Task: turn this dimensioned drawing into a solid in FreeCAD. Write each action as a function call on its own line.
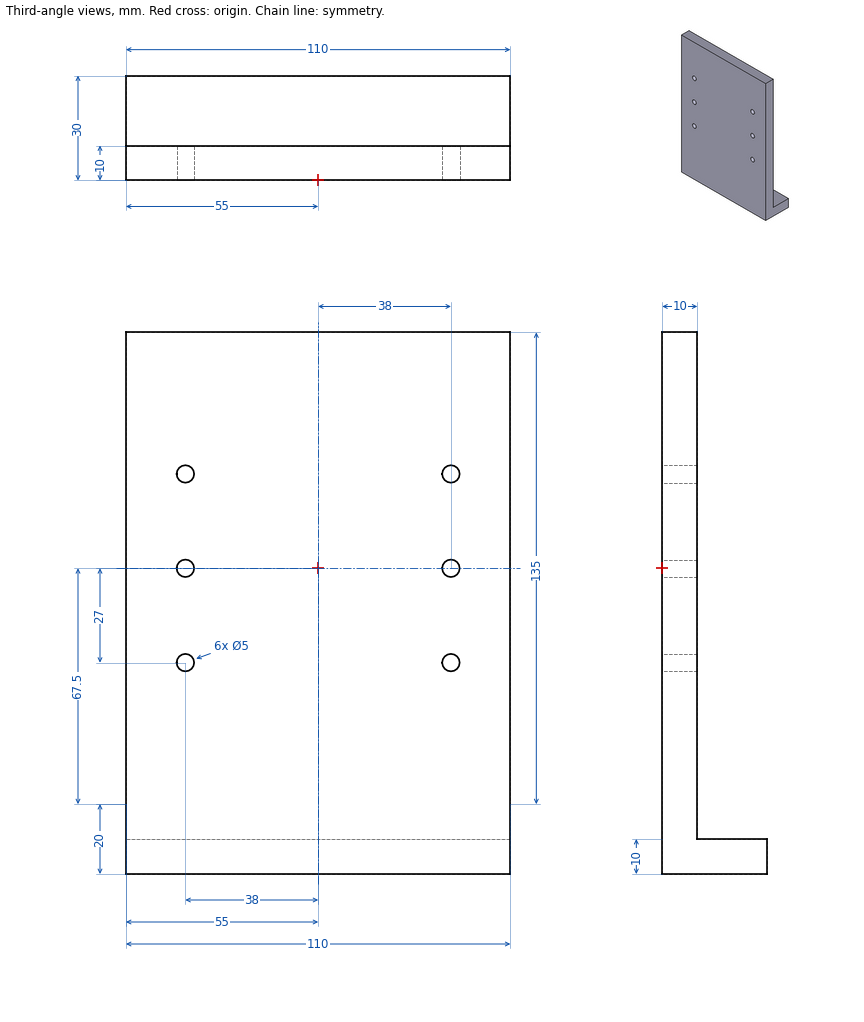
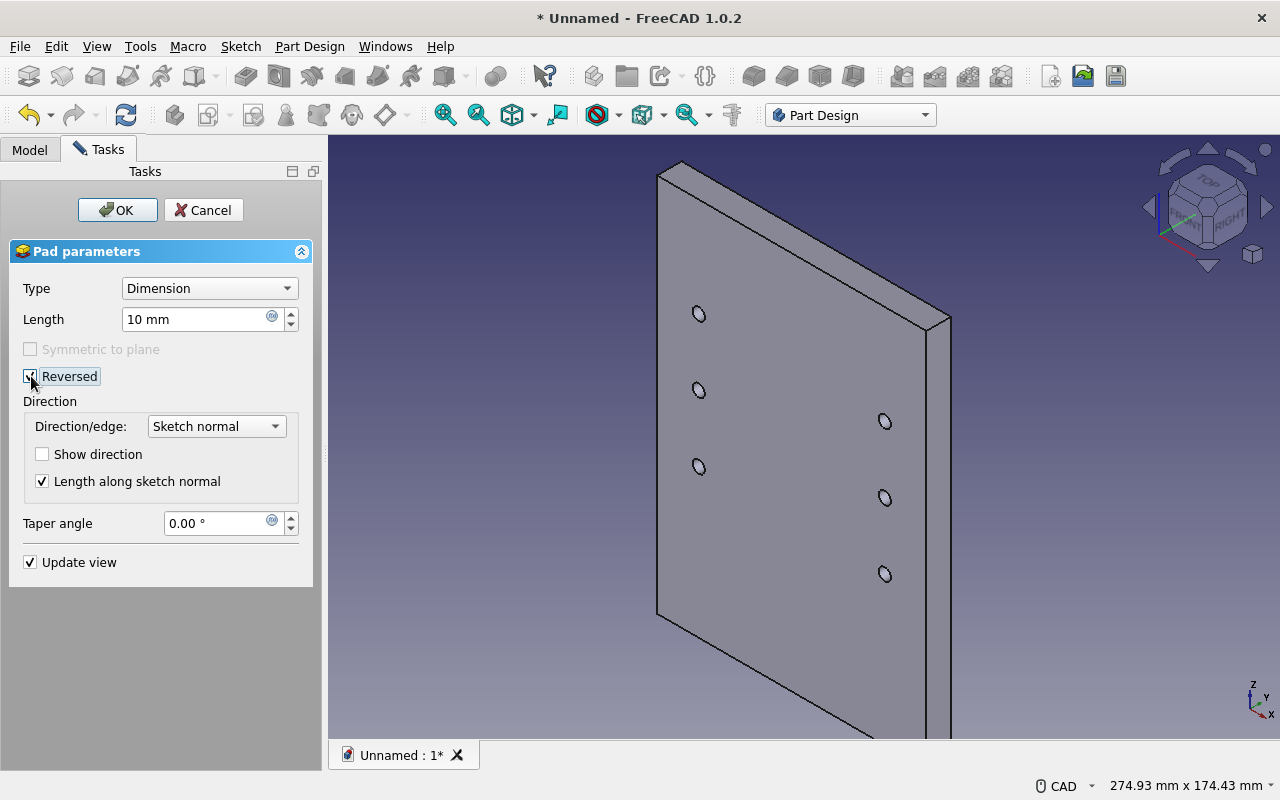
click(118, 210)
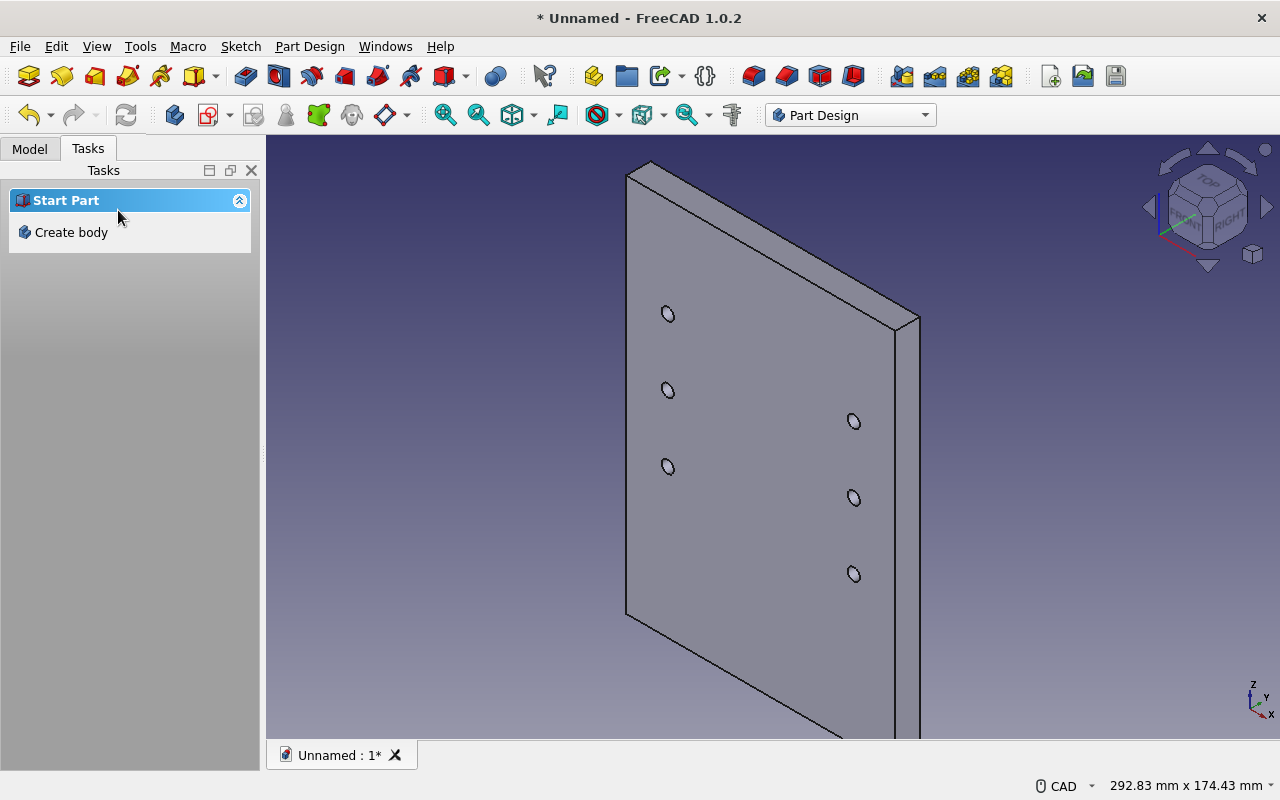
click(446, 116)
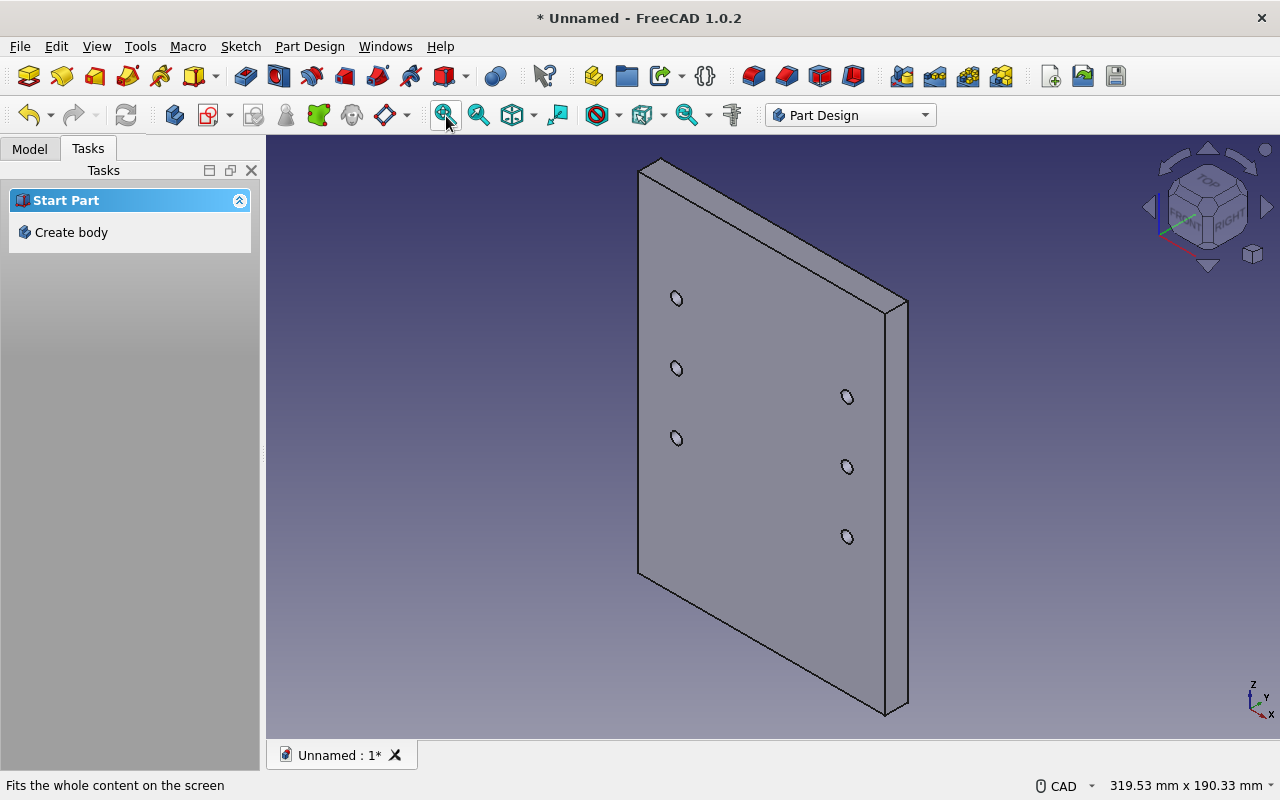
key(5)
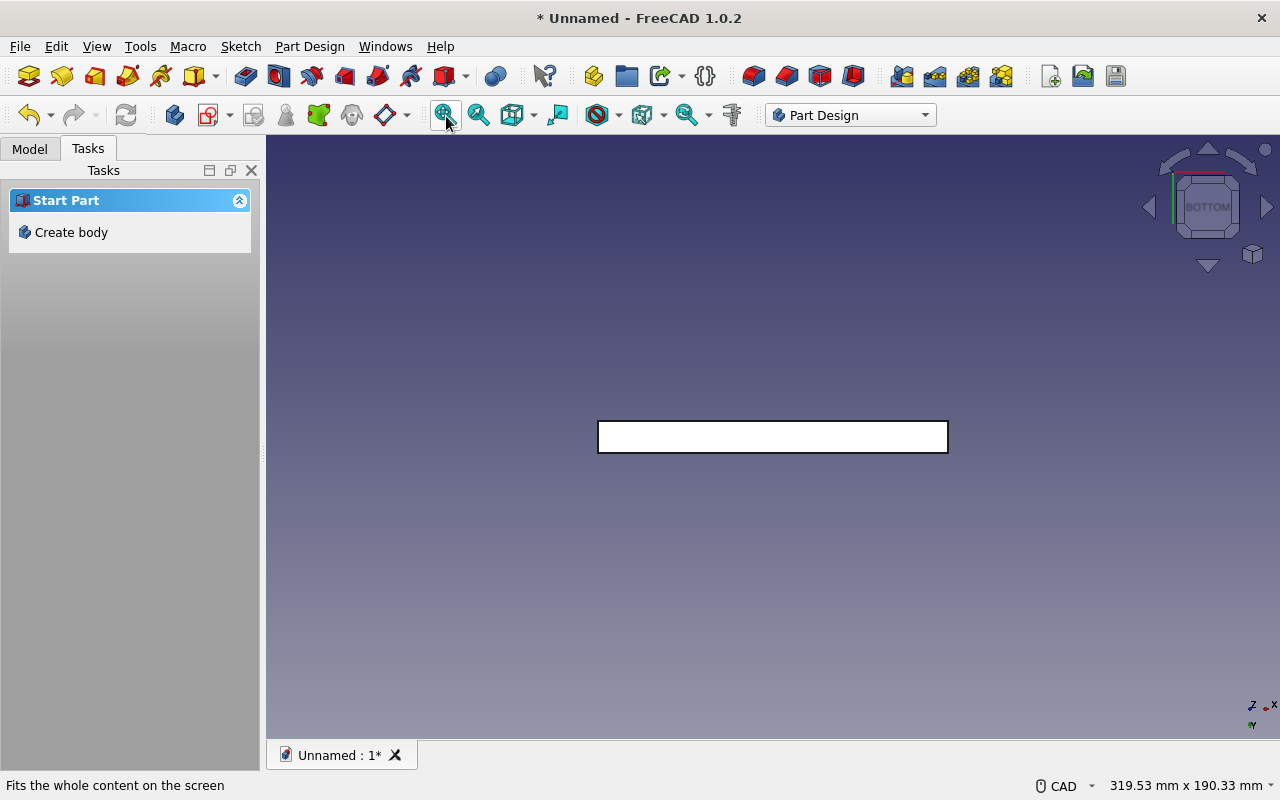
click(446, 116)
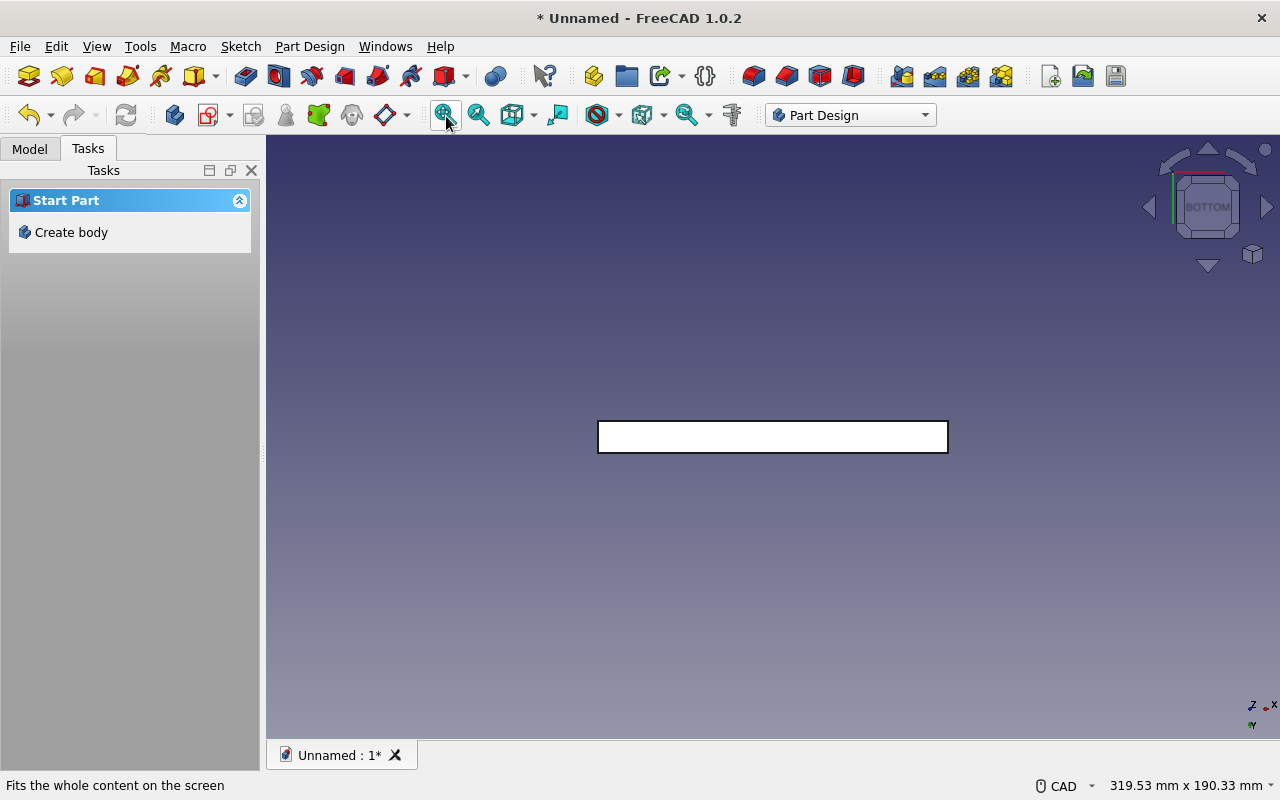
click(923, 436)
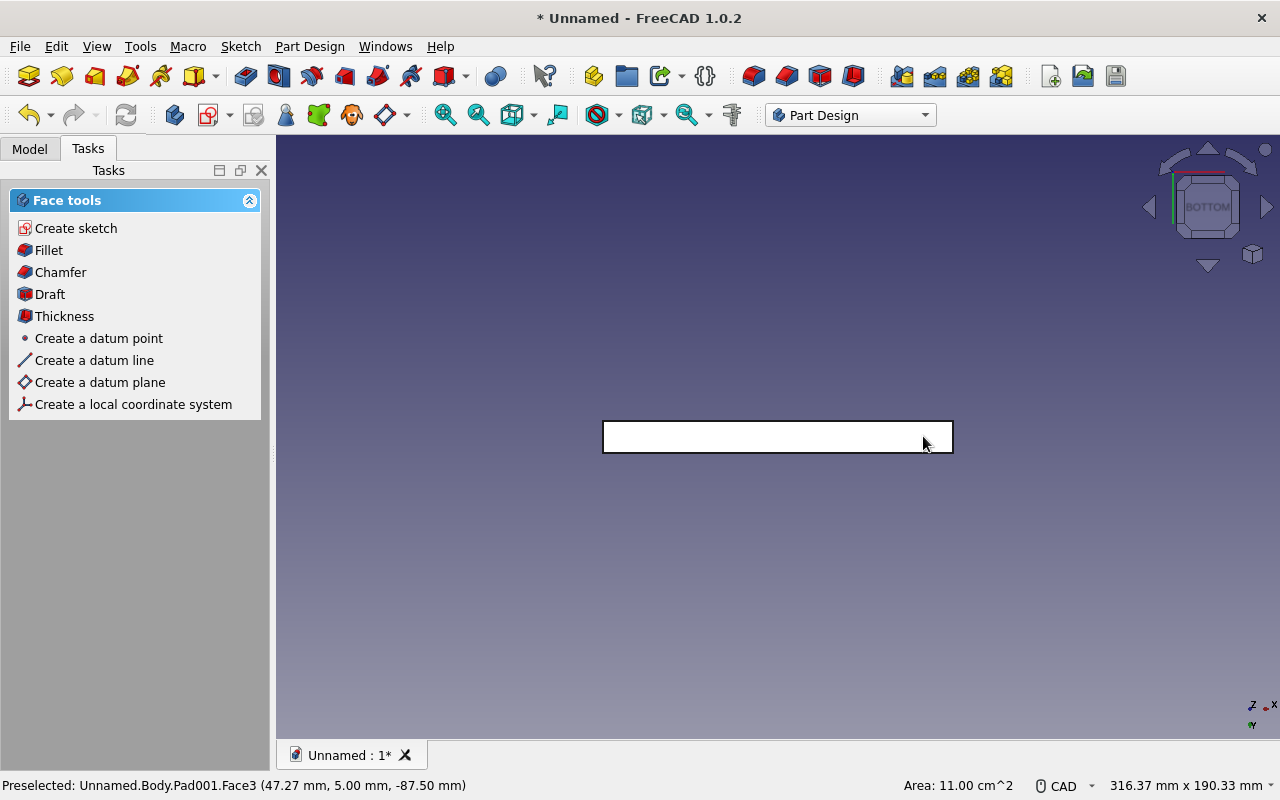
click(208, 116)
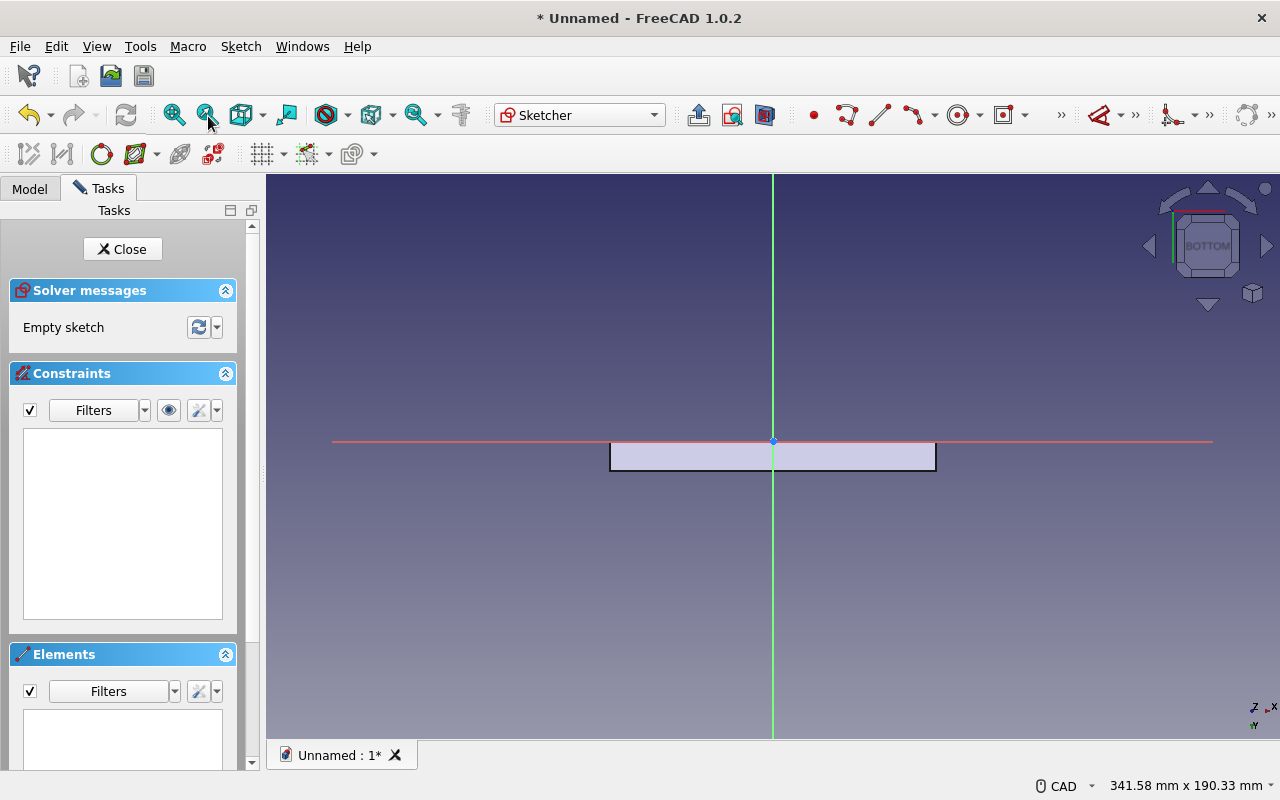
scroll(856, 522, up, 3)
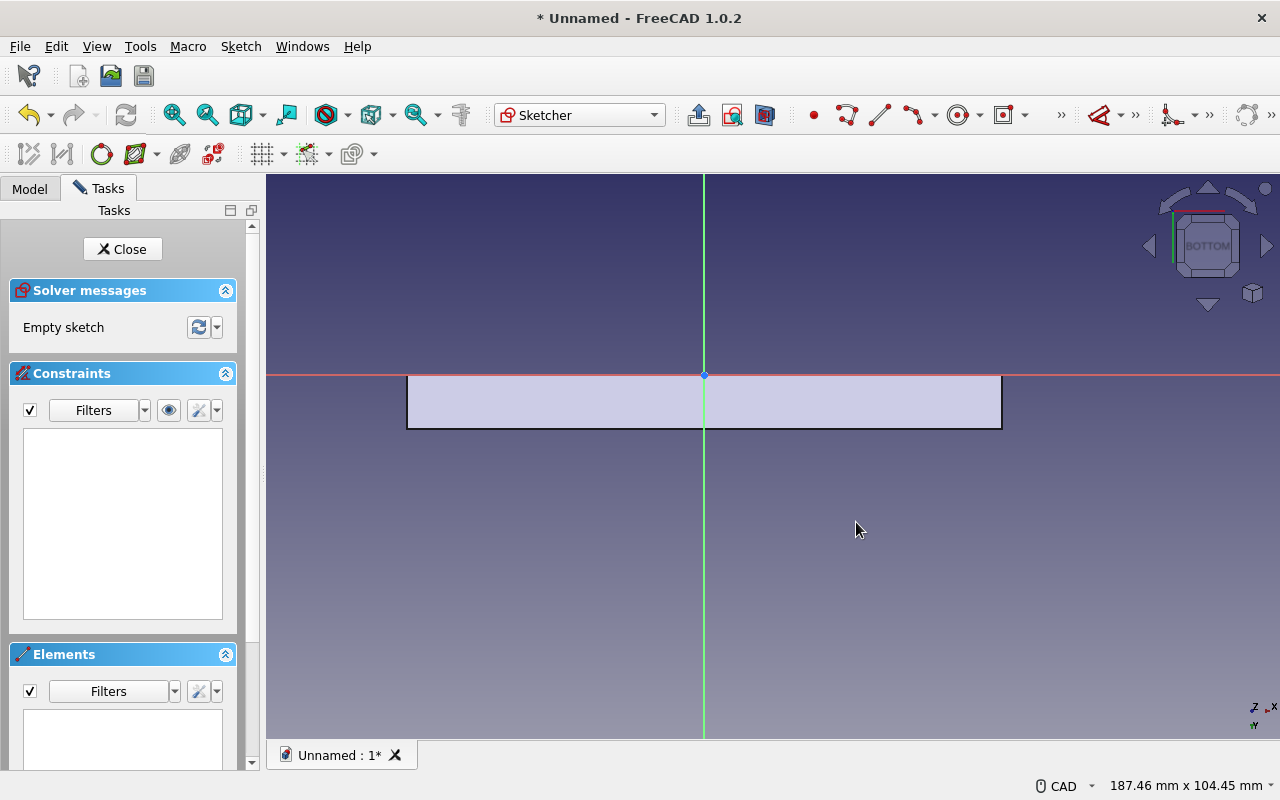
key(g)
key(r)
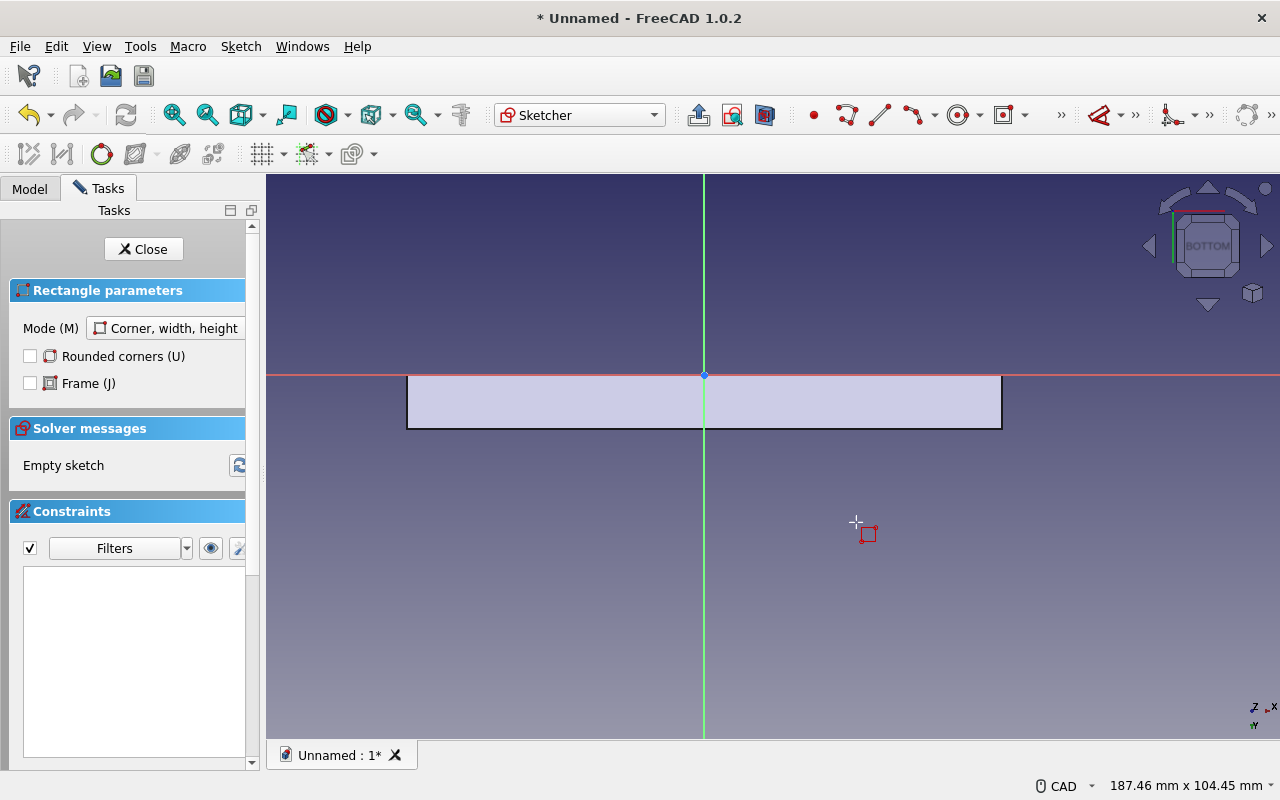
click(407, 375)
click(1002, 537)
key(Escape)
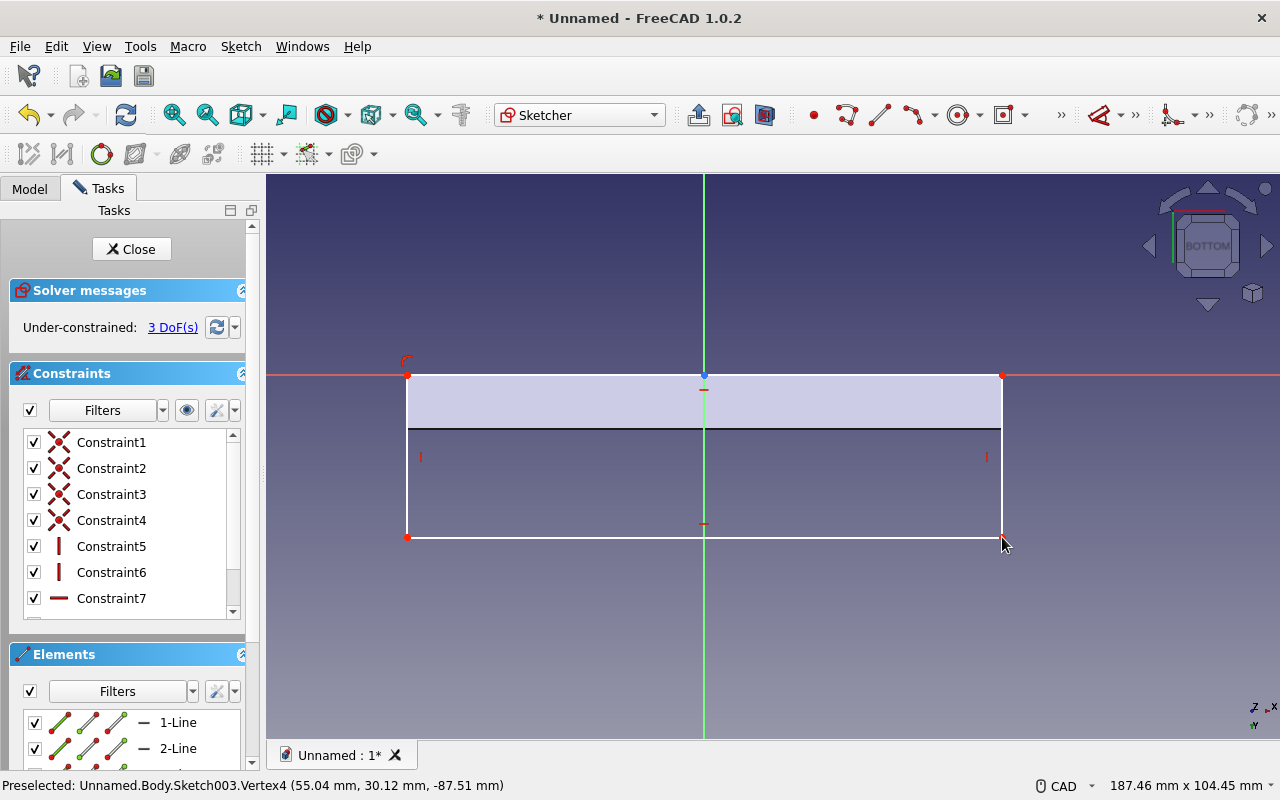
click(1098, 116)